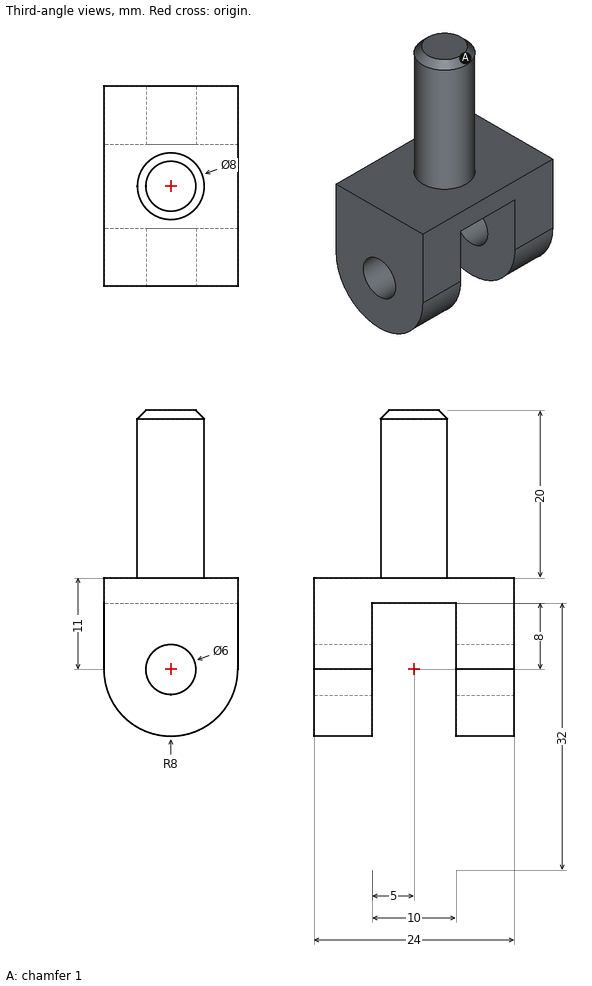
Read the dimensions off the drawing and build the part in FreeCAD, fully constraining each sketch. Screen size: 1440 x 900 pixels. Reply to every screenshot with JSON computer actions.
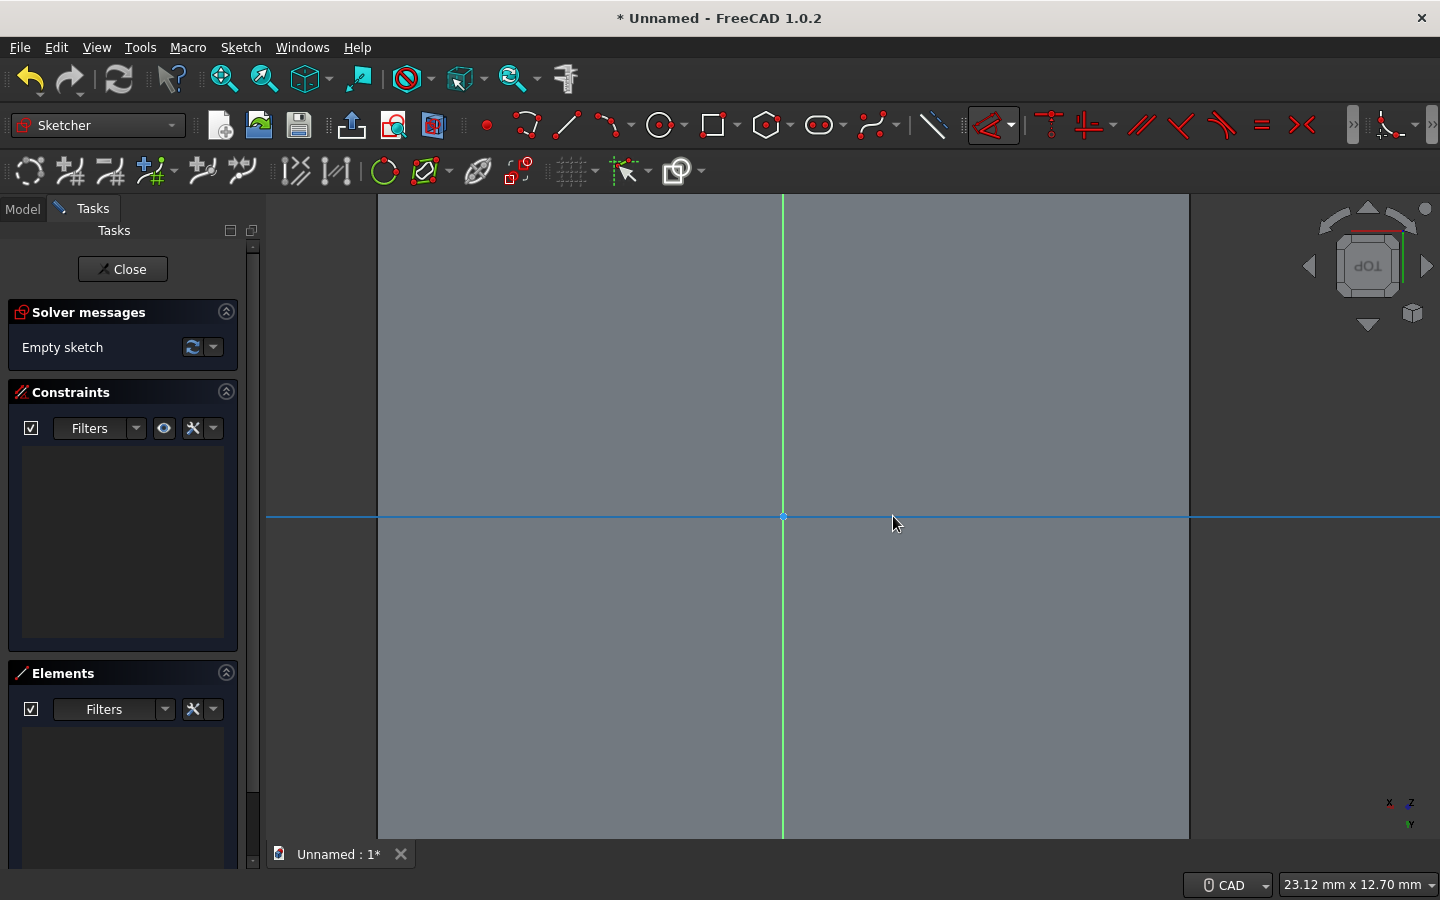
{"action": "left_click", "coordinate": [660, 126]}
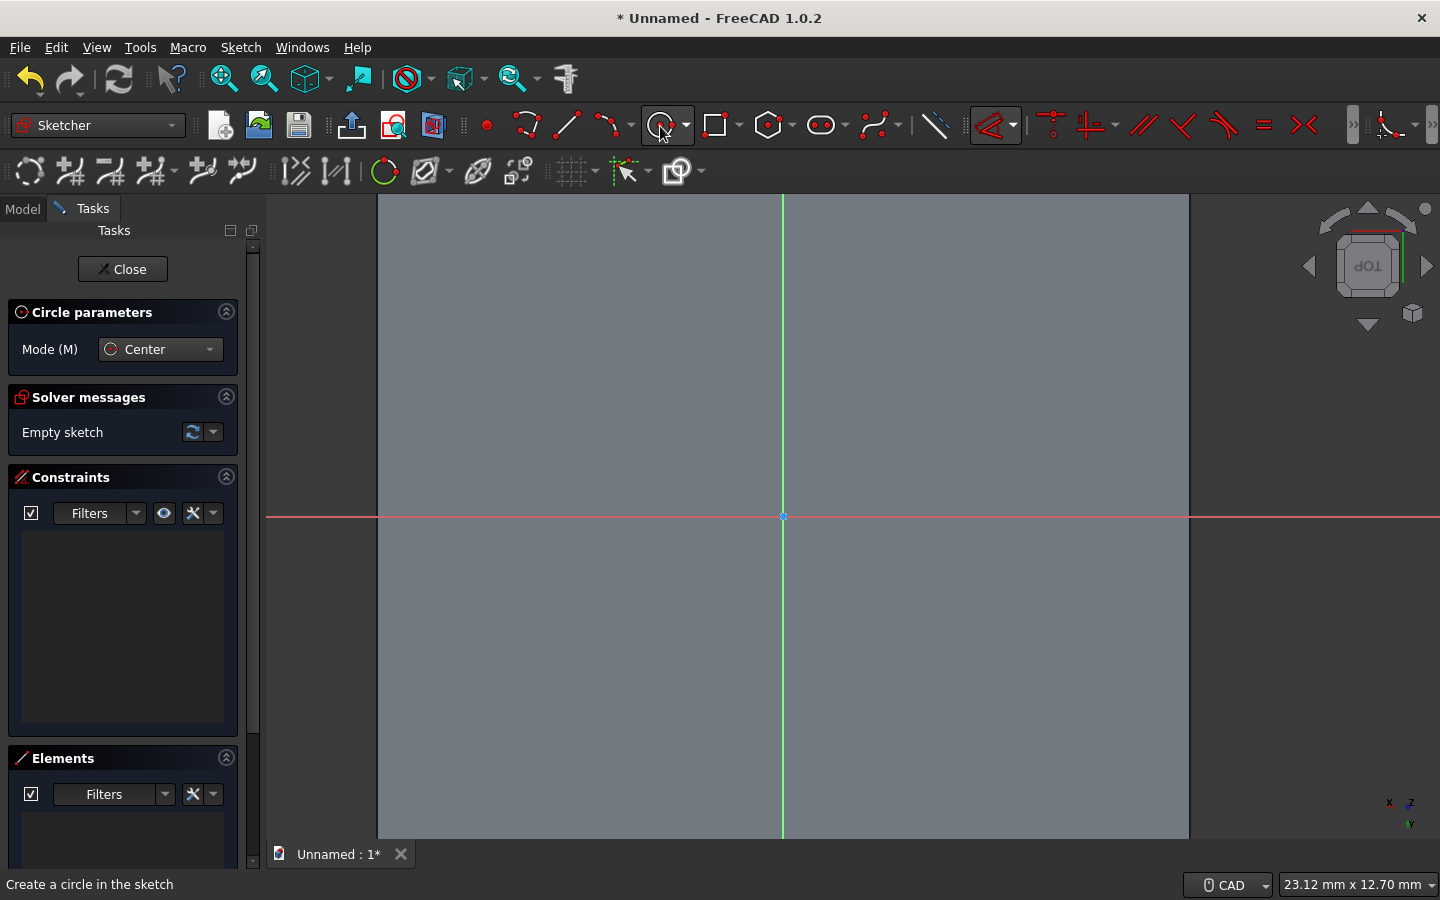
{"action": "left_click", "coordinate": [783, 517]}
{"action": "left_click", "coordinate": [927, 373]}
{"action": "key", "text": "Escape"}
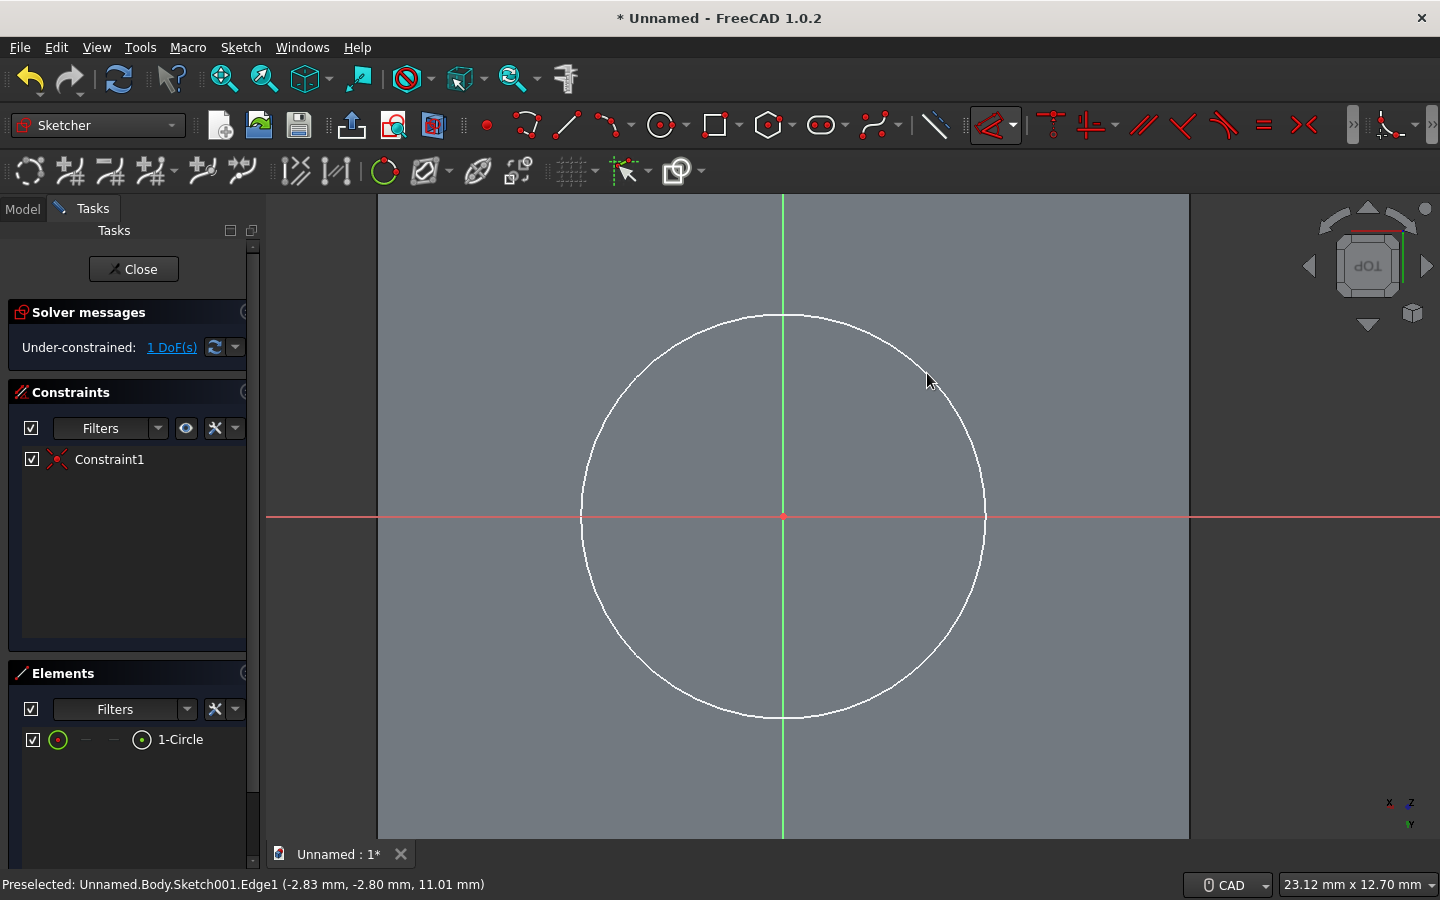
{"action": "left_click", "coordinate": [926, 373]}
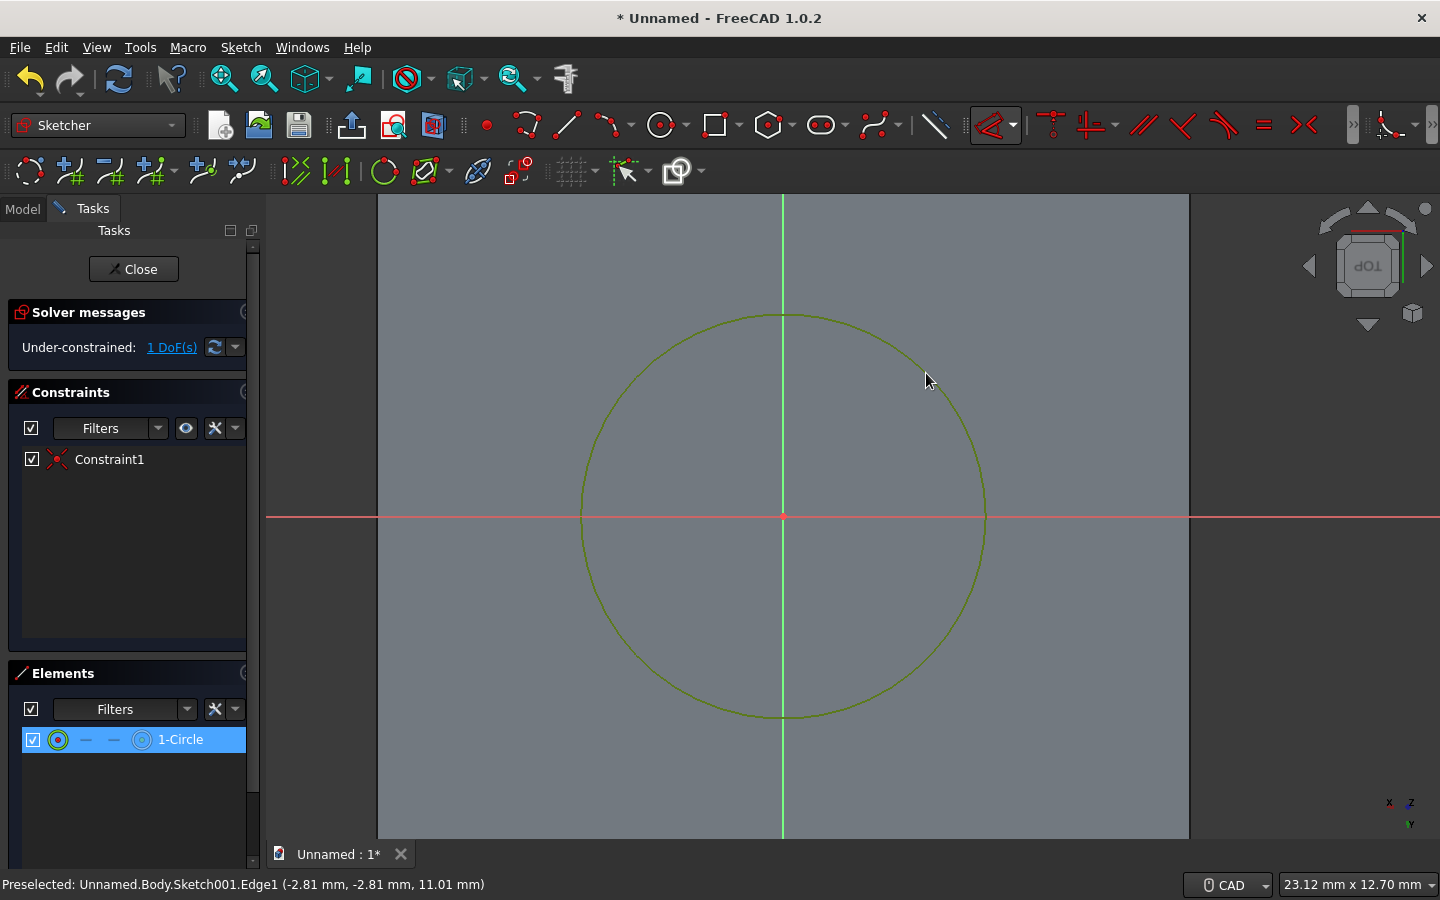
{"action": "key", "text": "k o"}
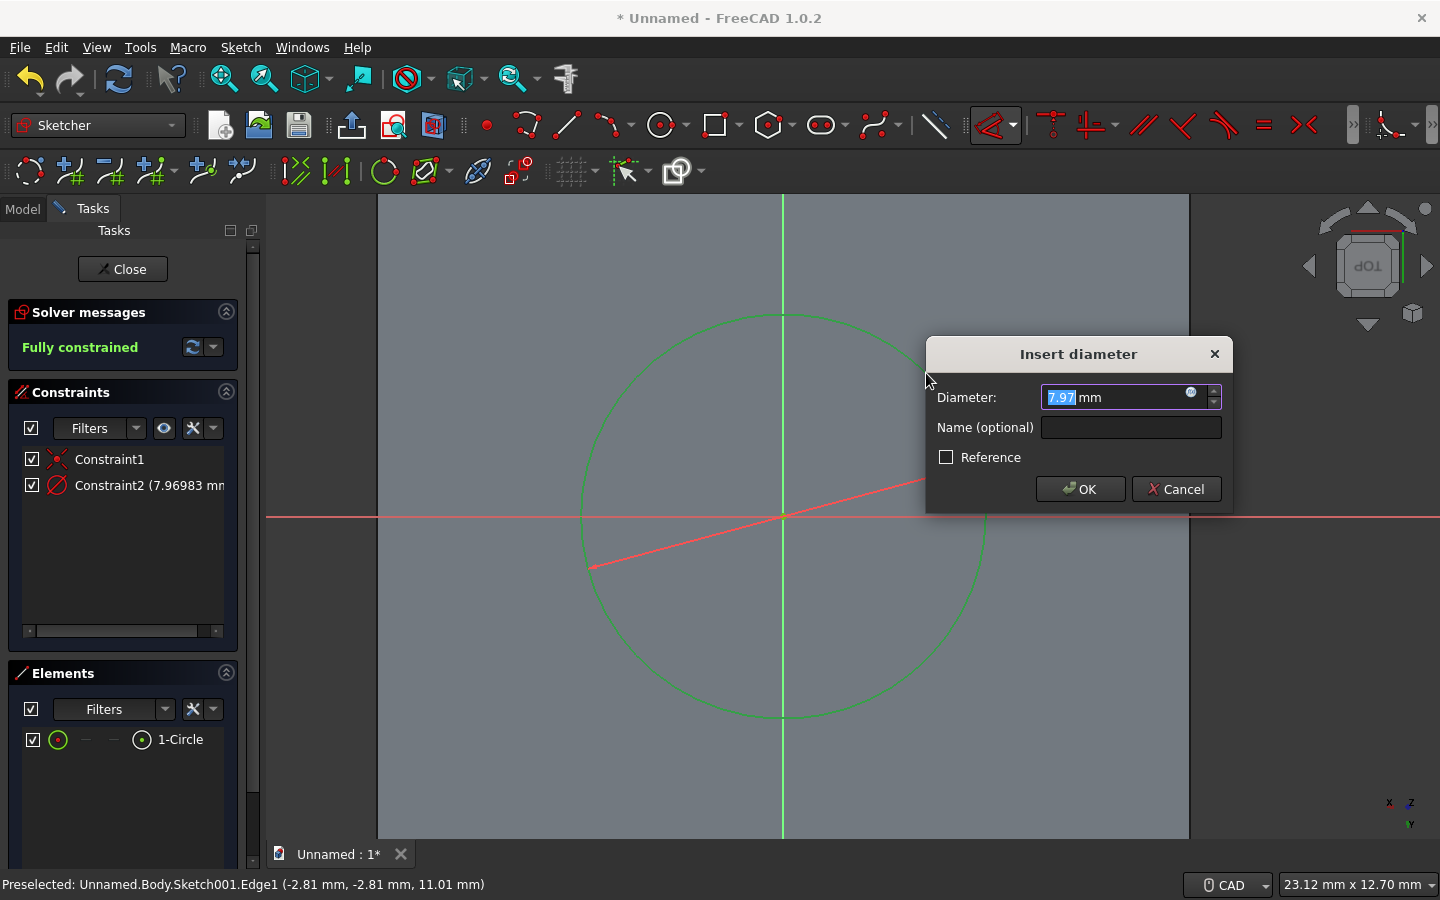
{"action": "type", "text": "8"}
{"action": "key", "text": "Return"}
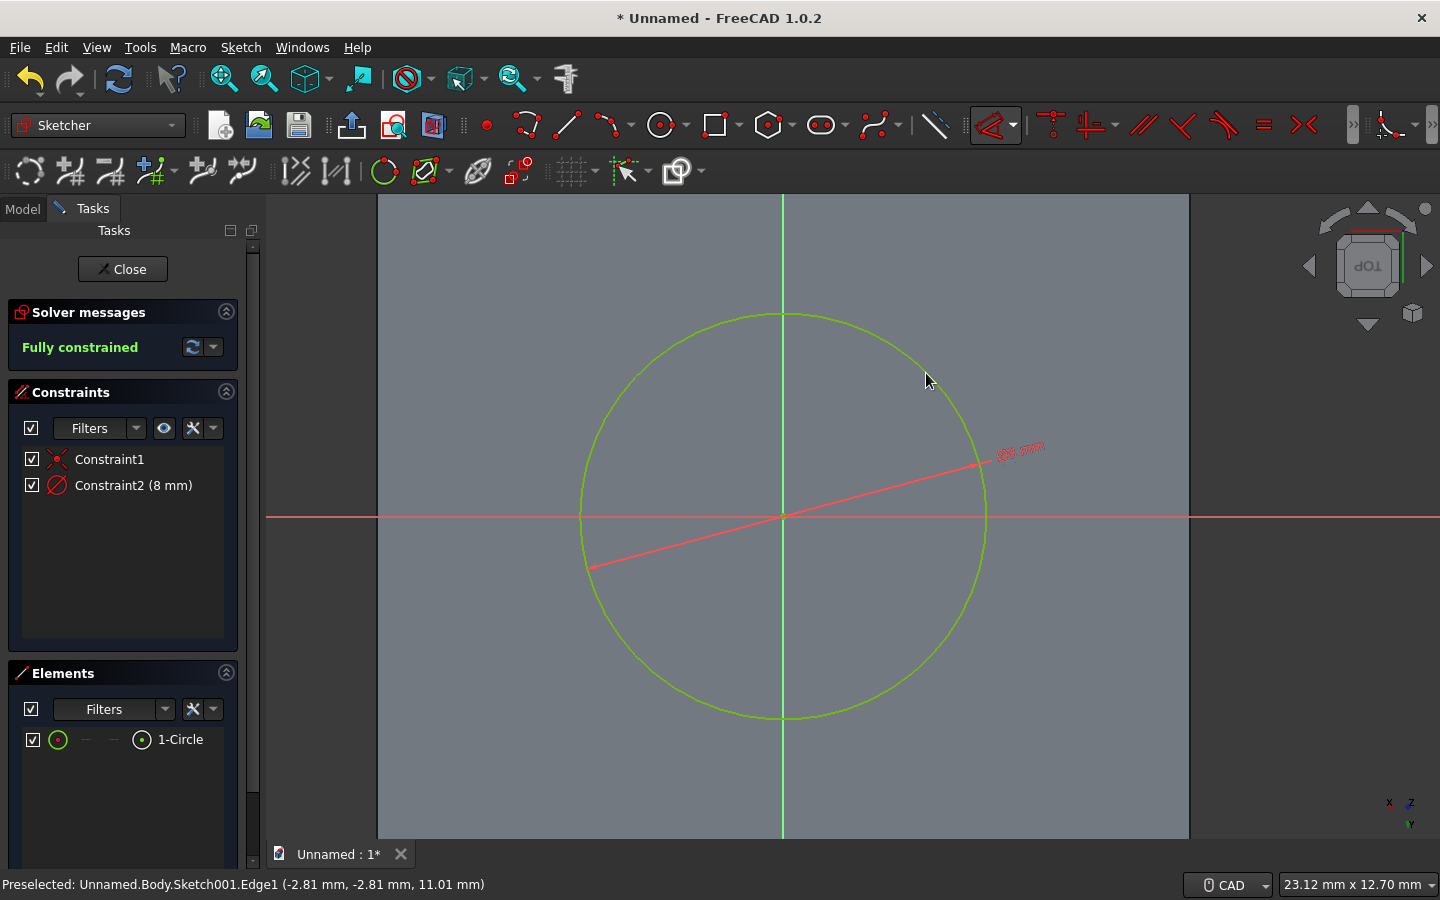
{"action": "left_click", "coordinate": [123, 269]}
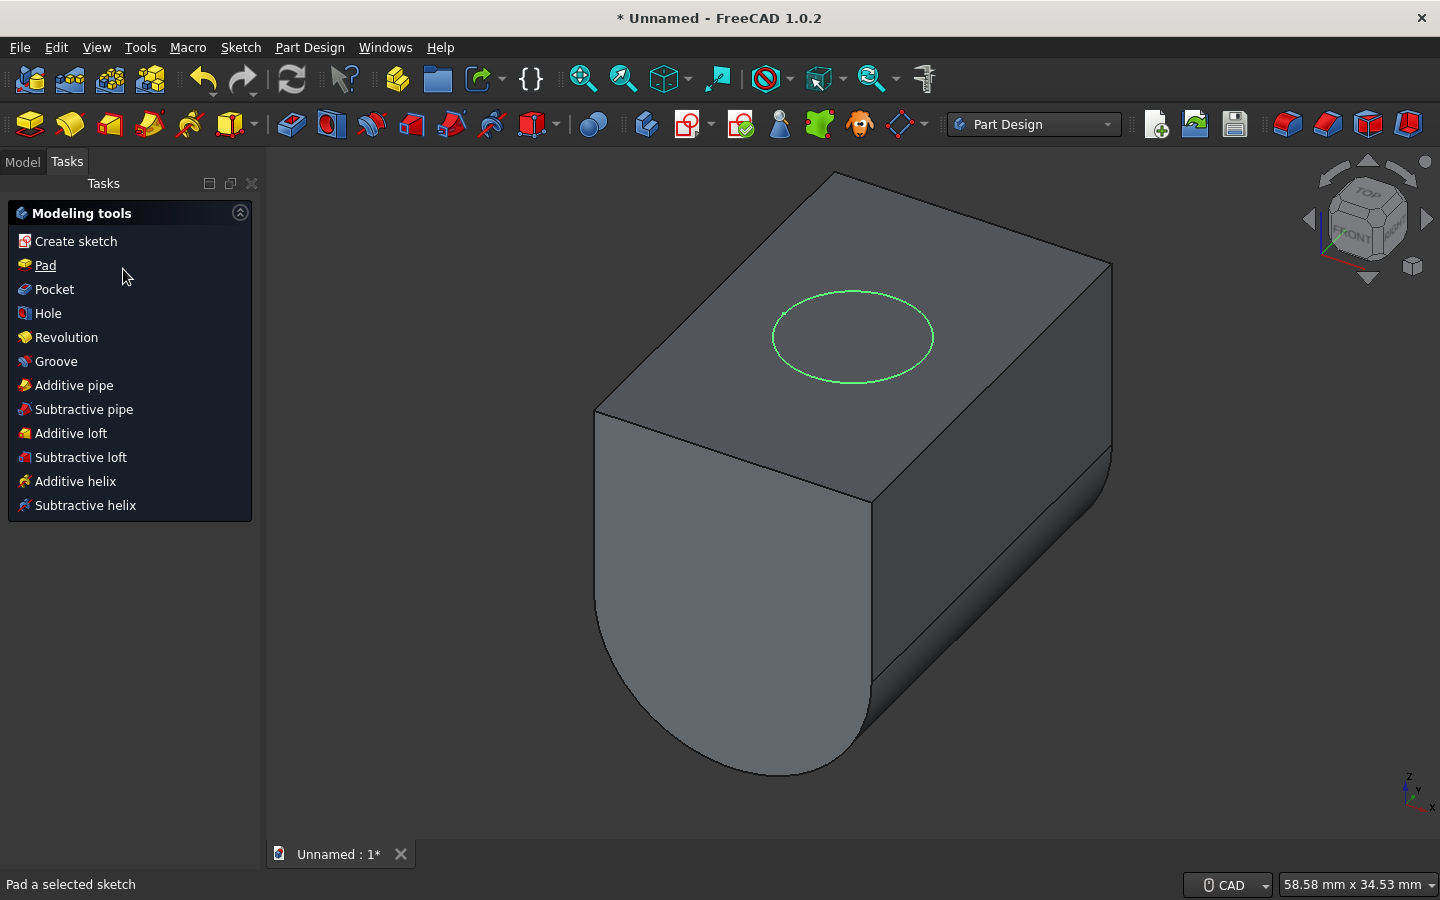
{"action": "left_click", "coordinate": [30, 124]}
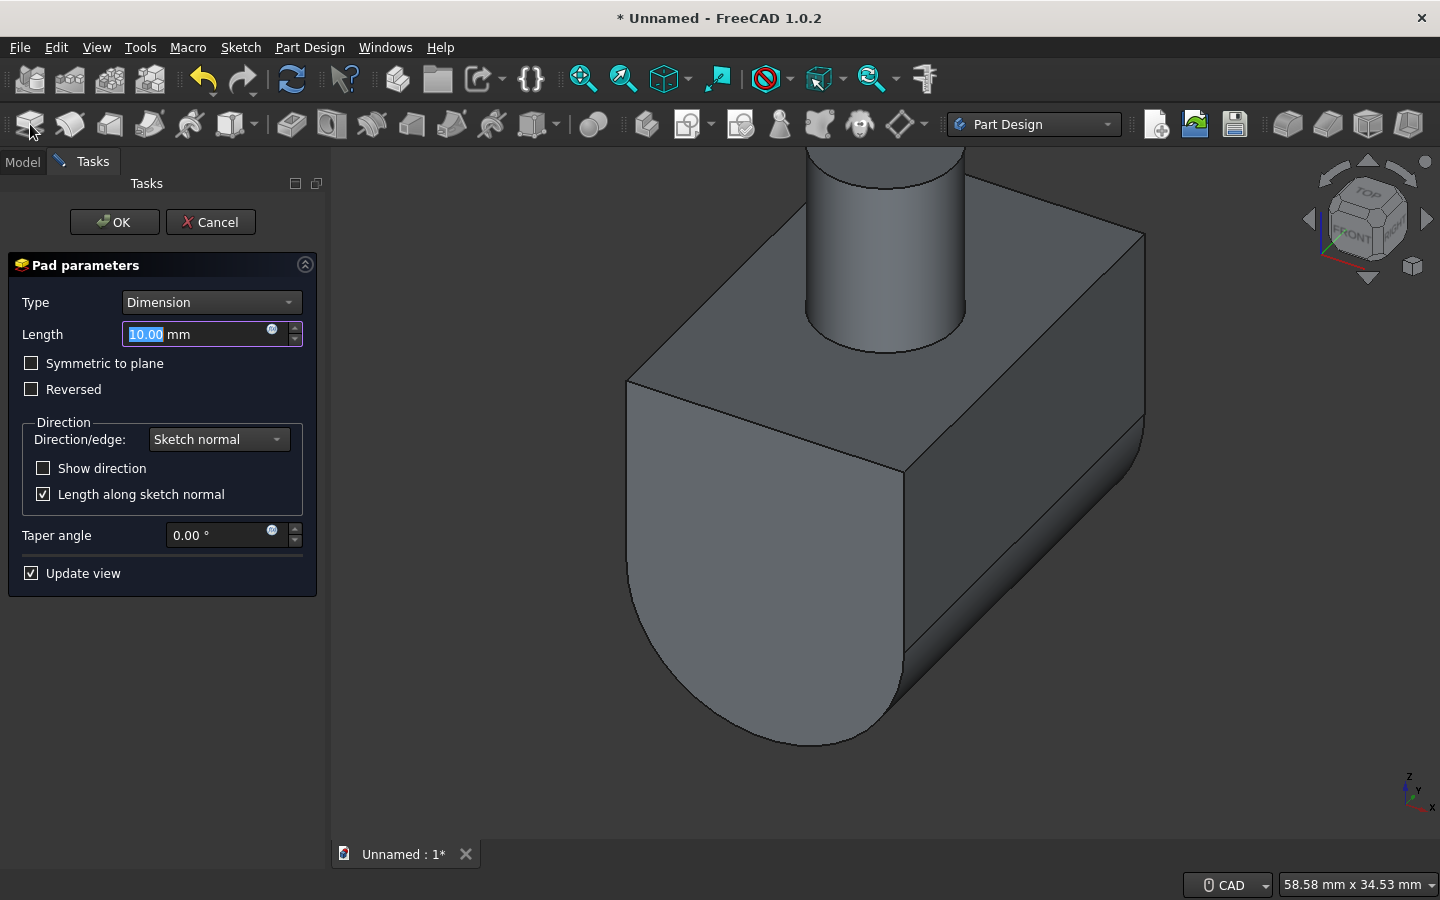
{"action": "type", "text": "20"}
{"action": "key", "text": "Tab"}